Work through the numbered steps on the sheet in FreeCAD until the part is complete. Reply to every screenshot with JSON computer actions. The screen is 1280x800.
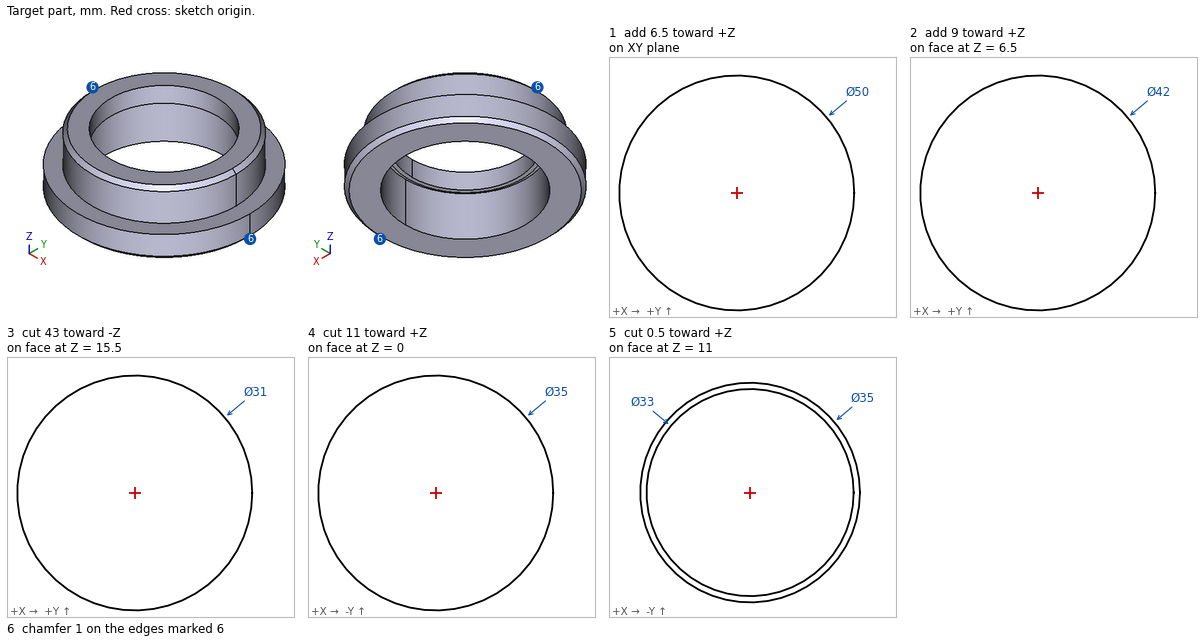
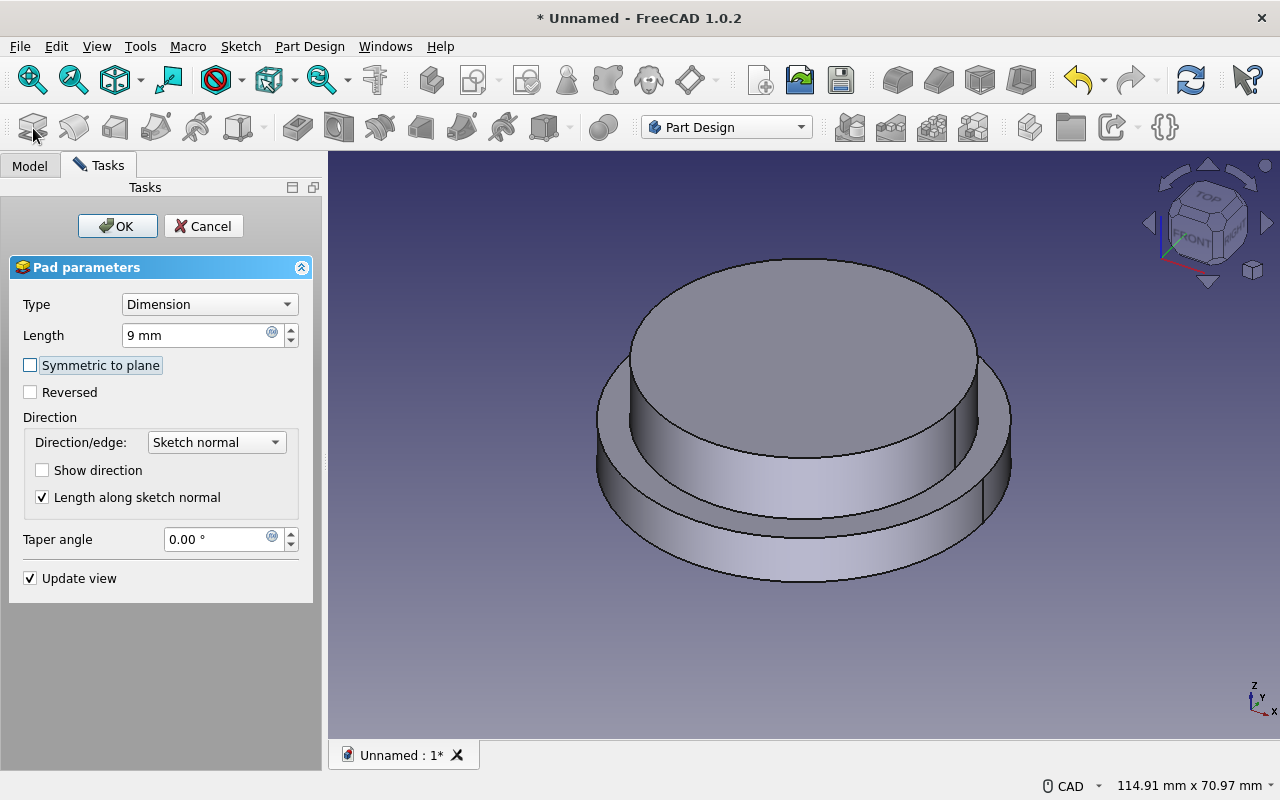
{"action": "left_click", "coordinate": [118, 226]}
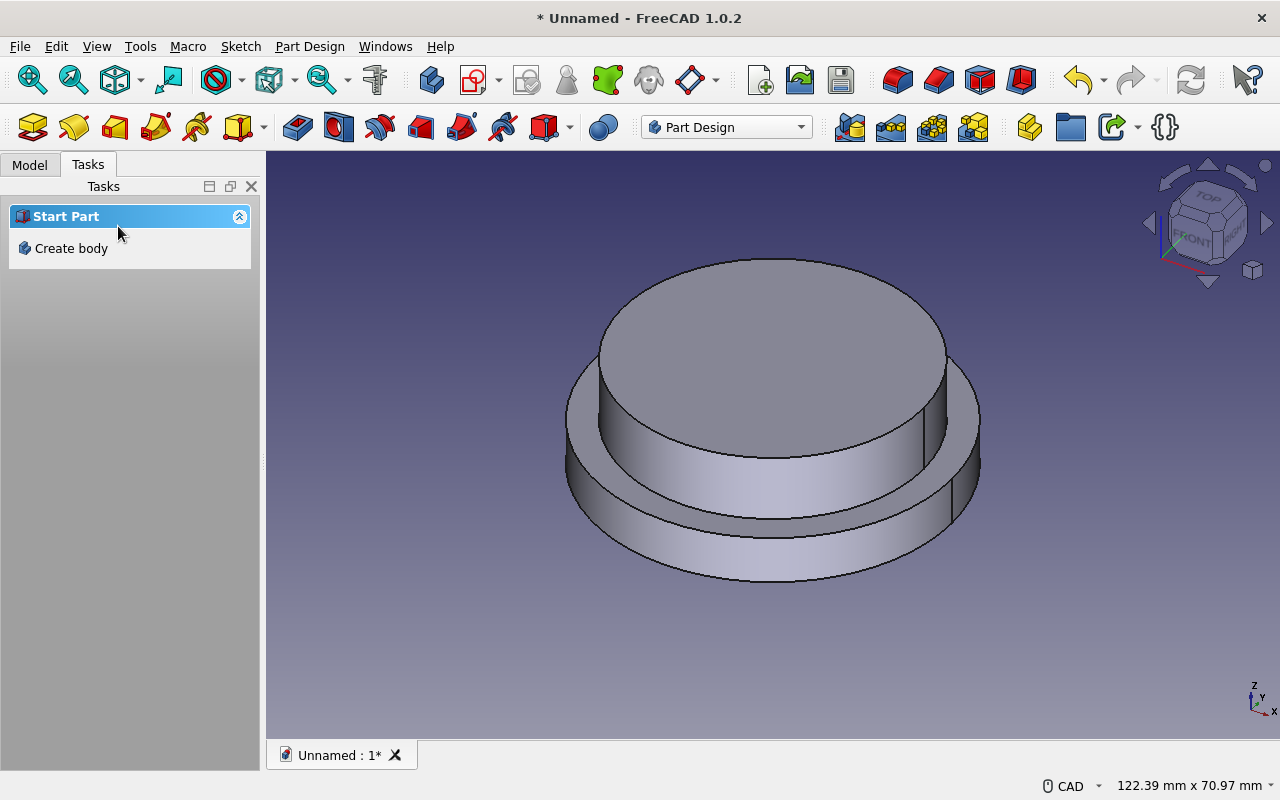
{"action": "left_click", "coordinate": [773, 357]}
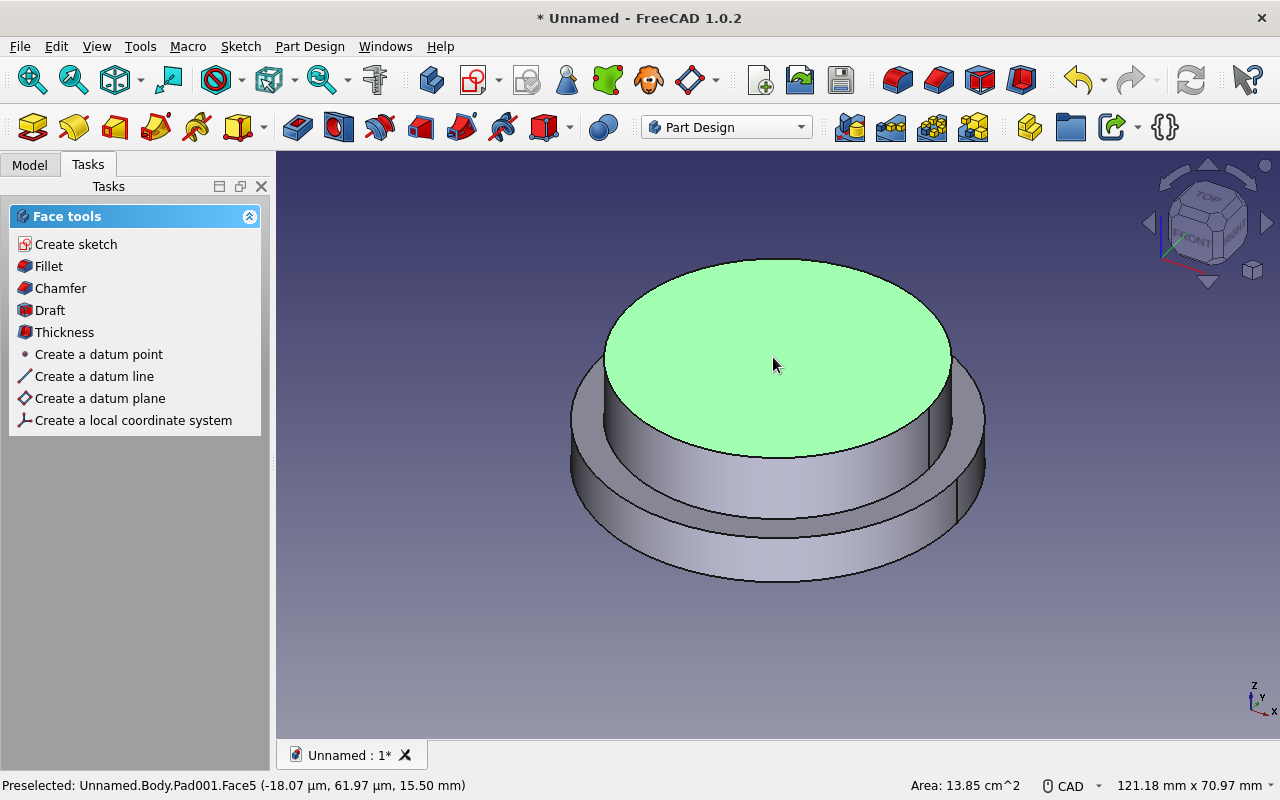
{"action": "left_click", "coordinate": [472, 80]}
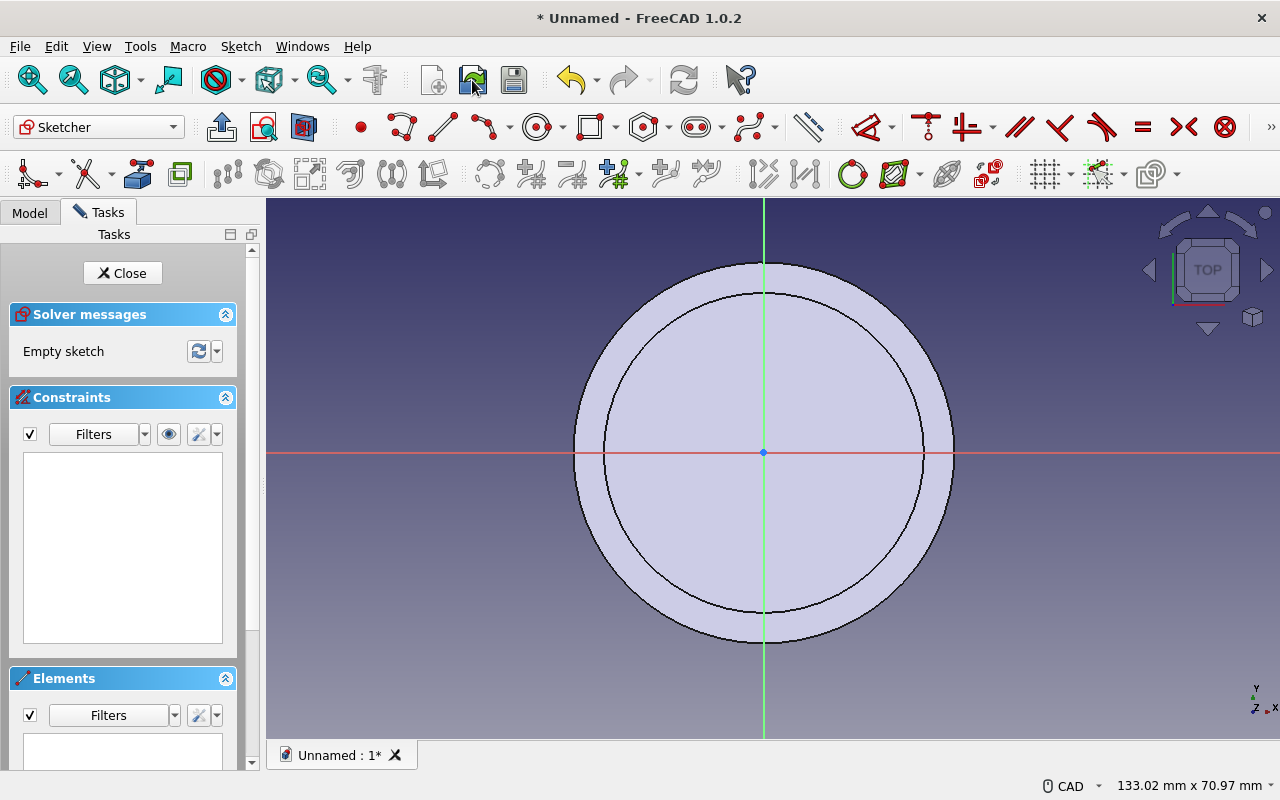
{"action": "scroll", "coordinate": [885, 421], "scroll_direction": "up", "scroll_amount": 2}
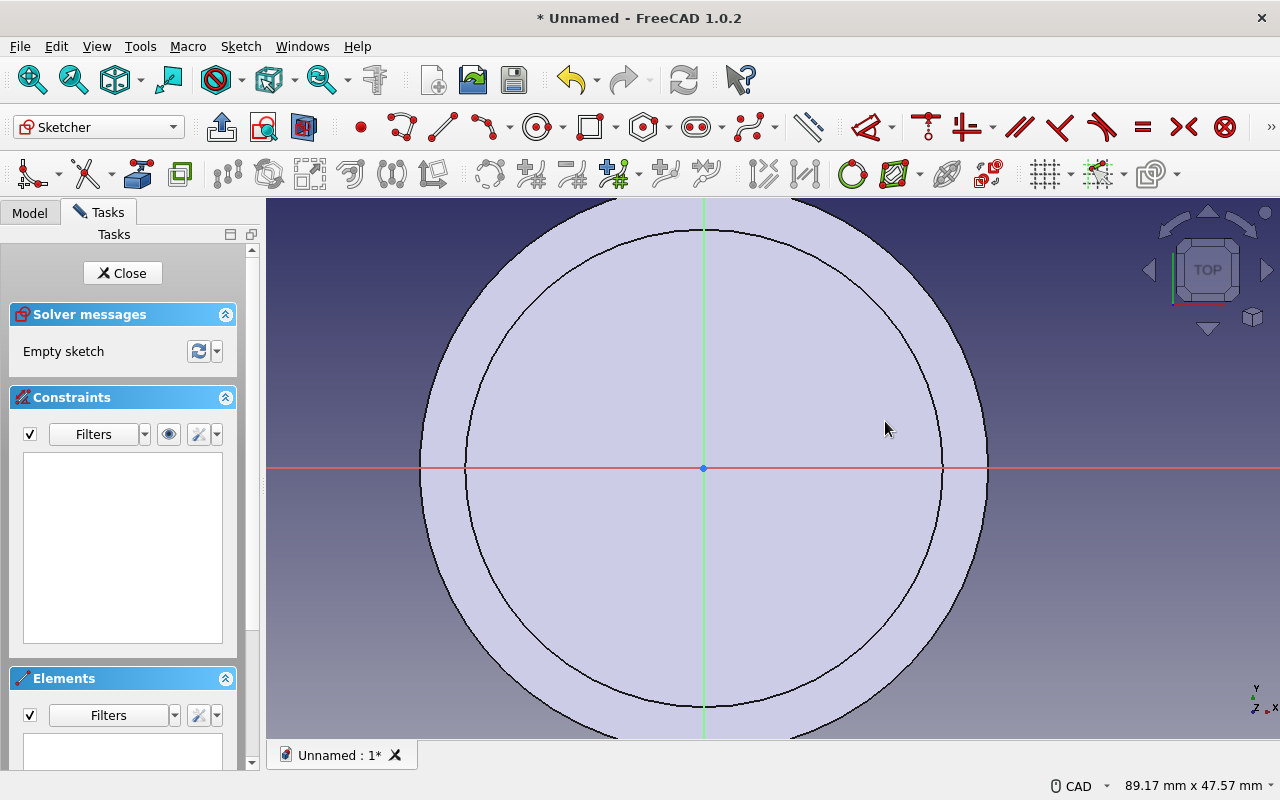
{"action": "left_click", "coordinate": [536, 128]}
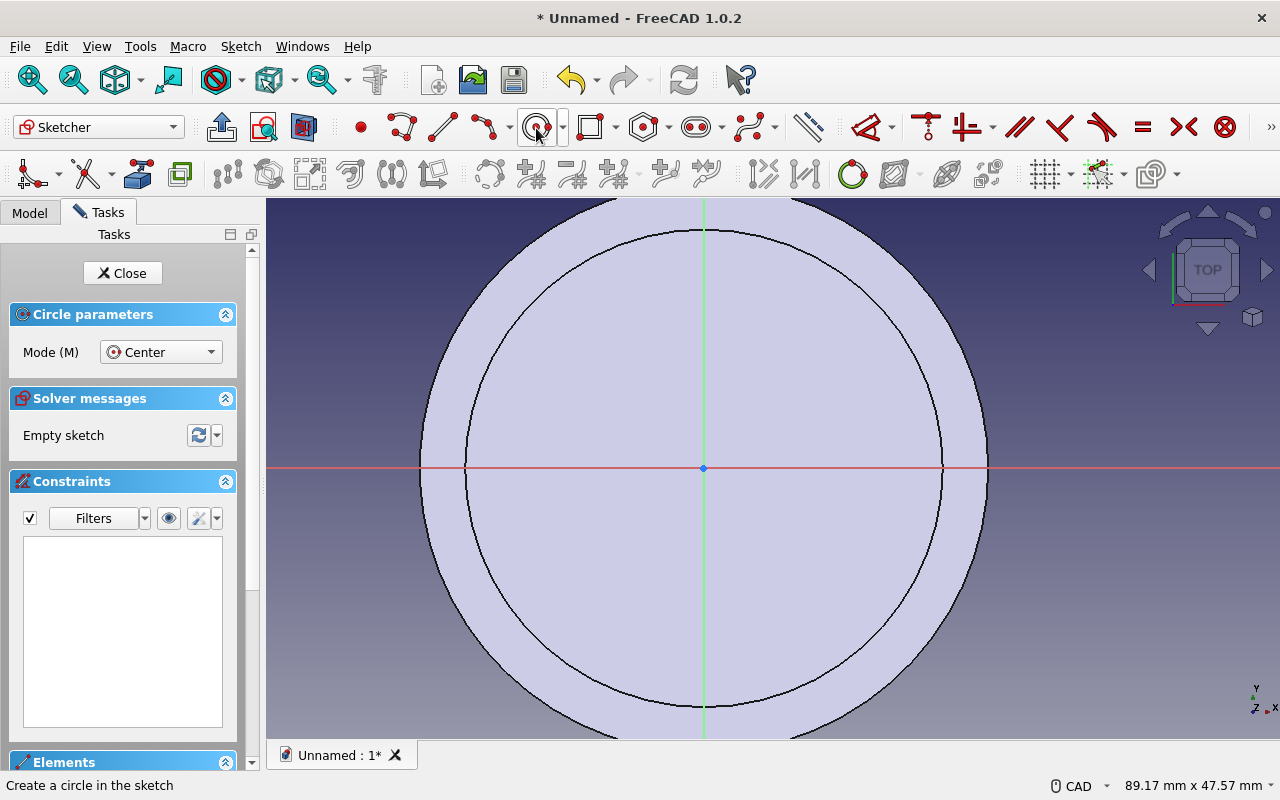
{"action": "left_click", "coordinate": [704, 468]}
{"action": "mouse_move", "coordinate": [829, 344]}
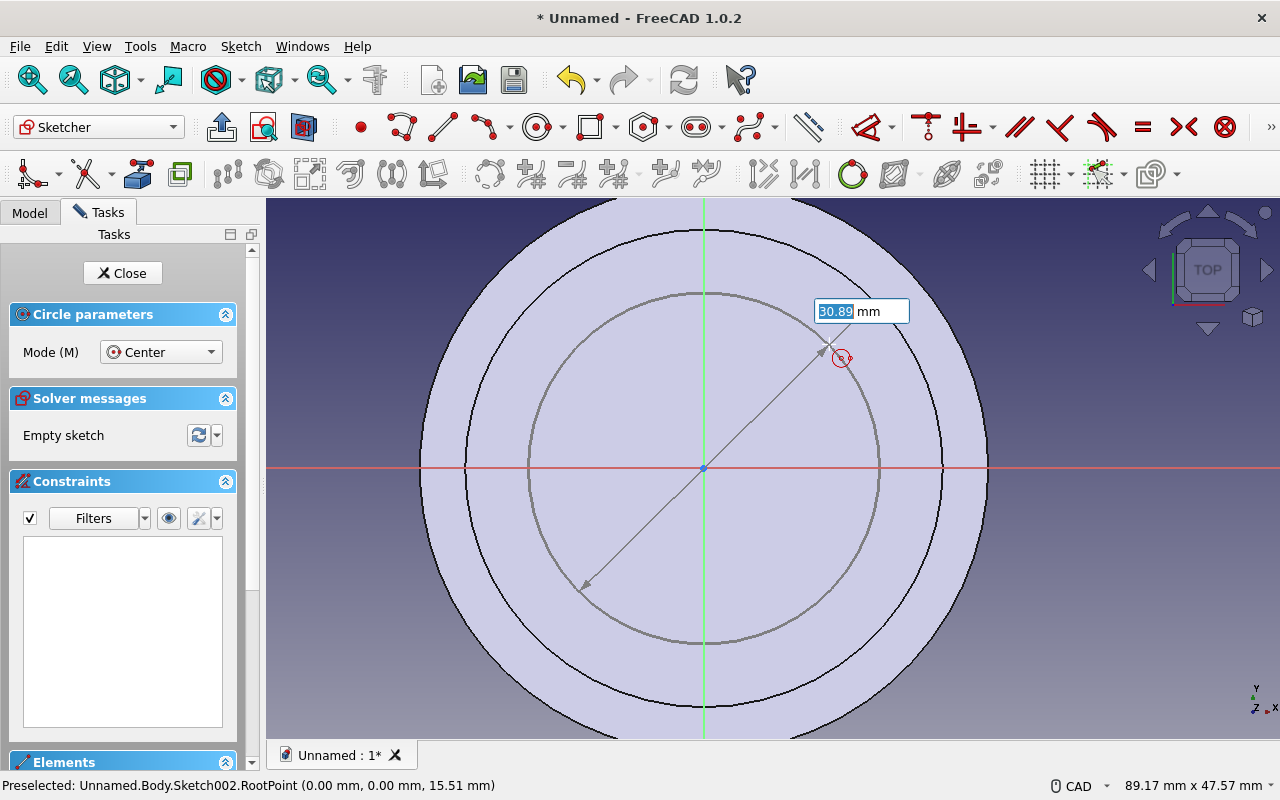
{"action": "type", "text": "31"}
{"action": "key", "text": "Return"}
{"action": "key", "text": "Escape"}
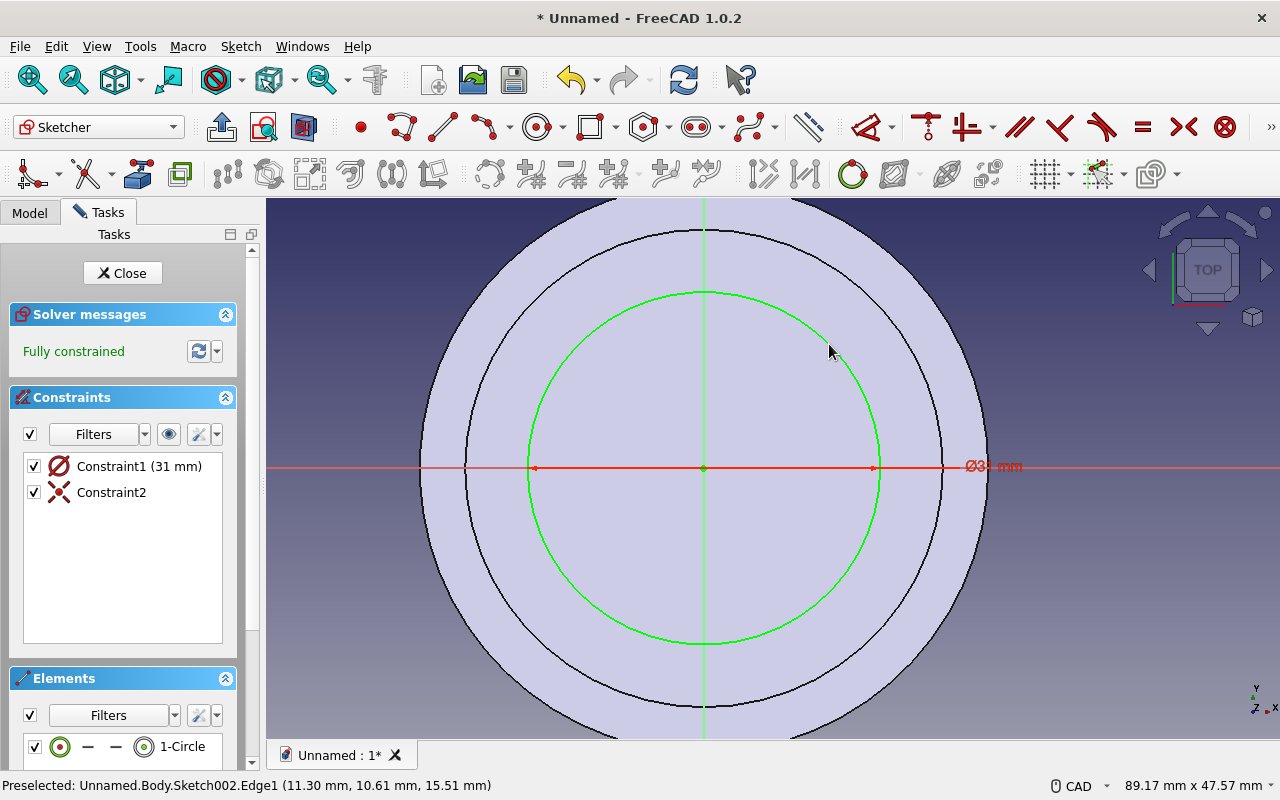
{"action": "left_click", "coordinate": [123, 273]}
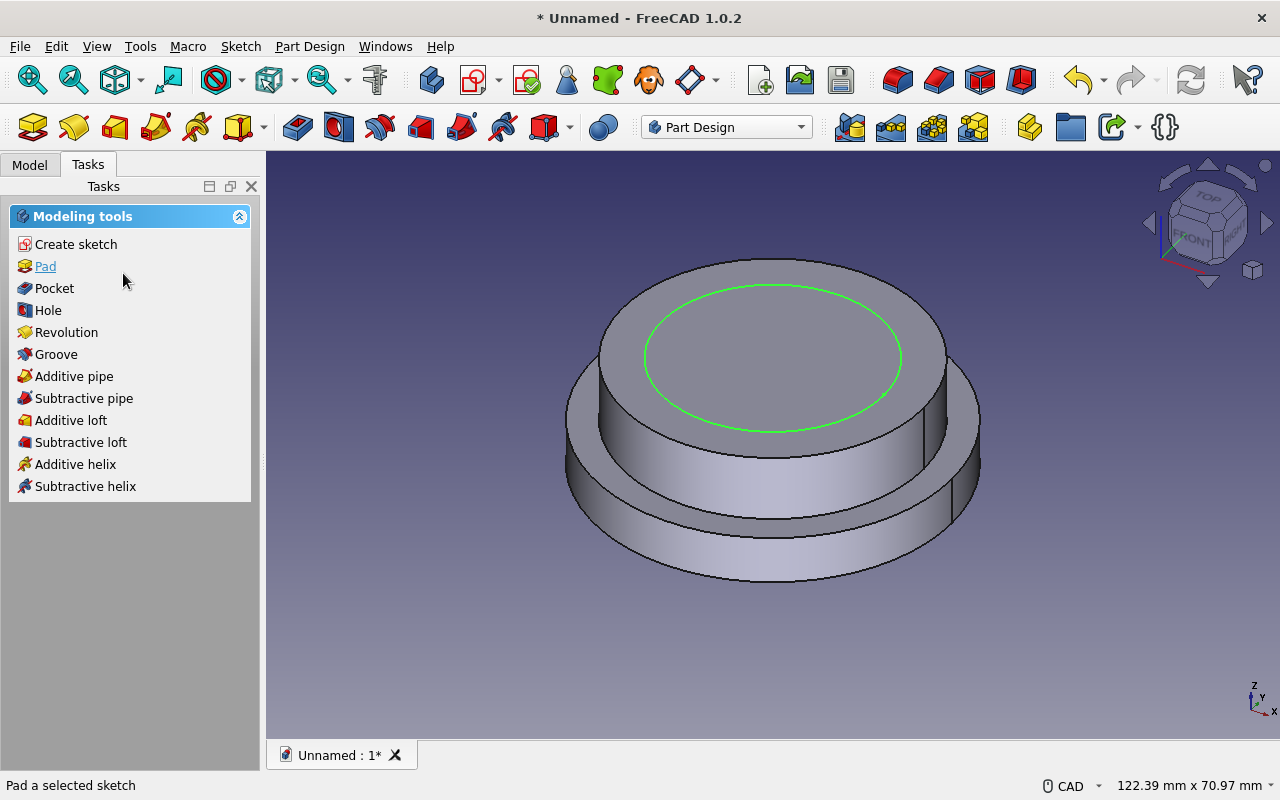
{"action": "left_click", "coordinate": [298, 128]}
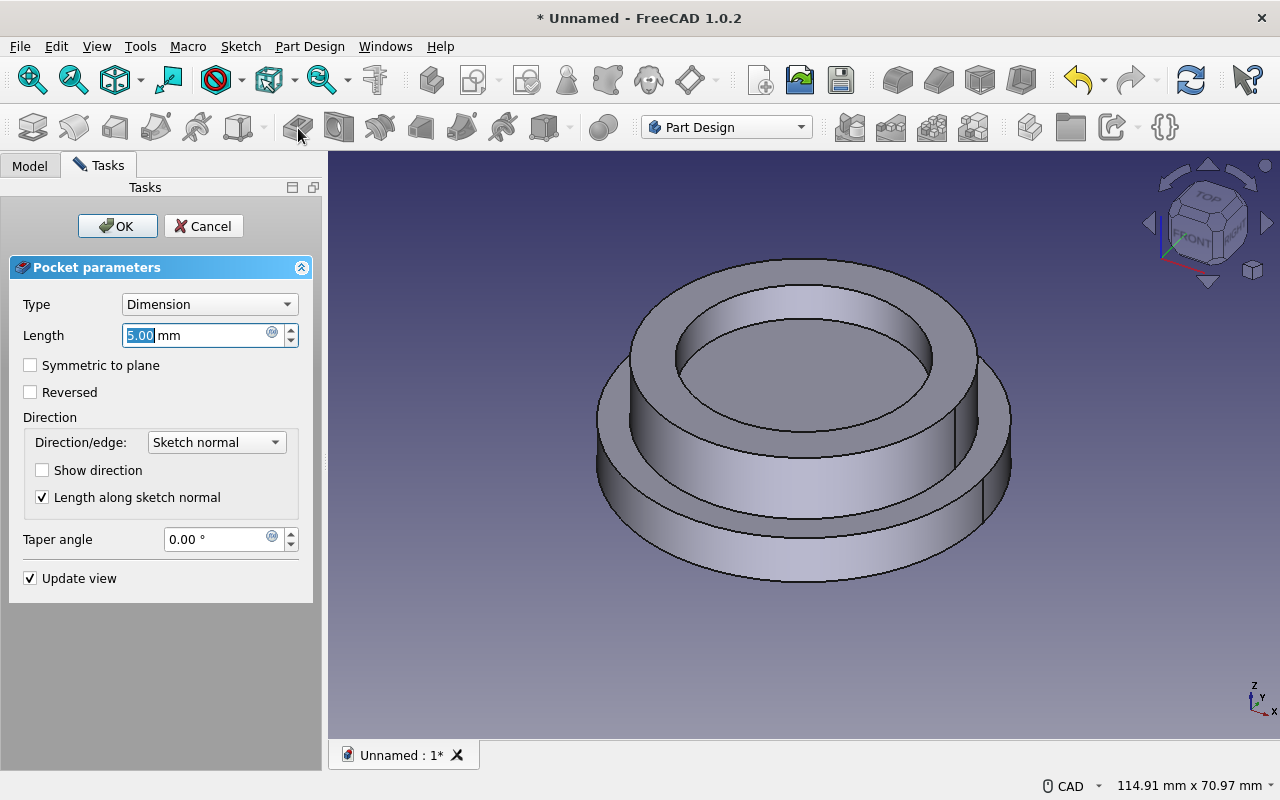
{"action": "type", "text": "43"}
{"action": "key", "text": "Tab"}